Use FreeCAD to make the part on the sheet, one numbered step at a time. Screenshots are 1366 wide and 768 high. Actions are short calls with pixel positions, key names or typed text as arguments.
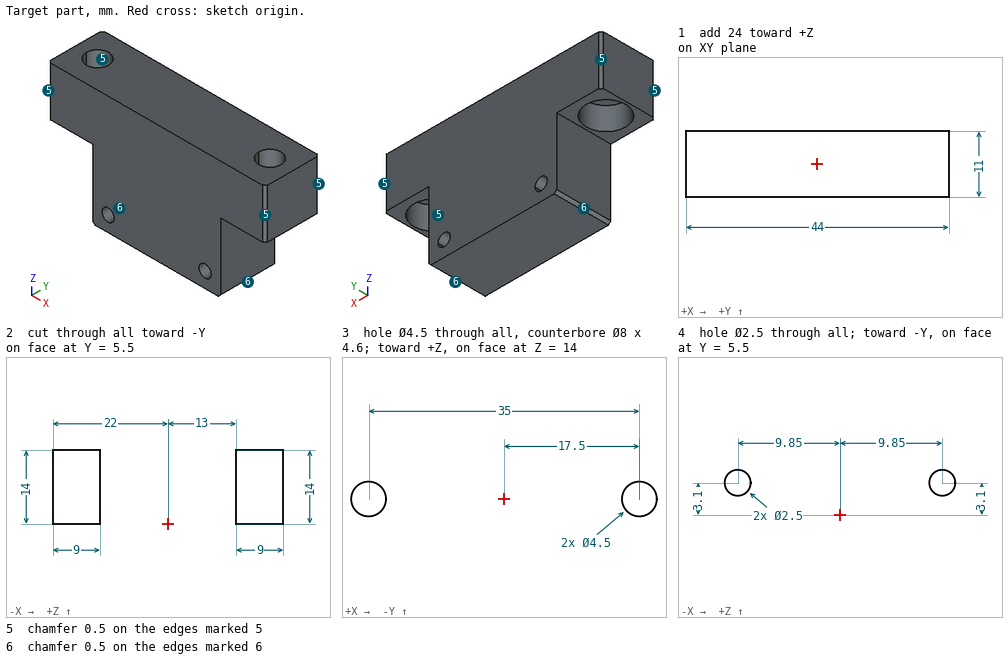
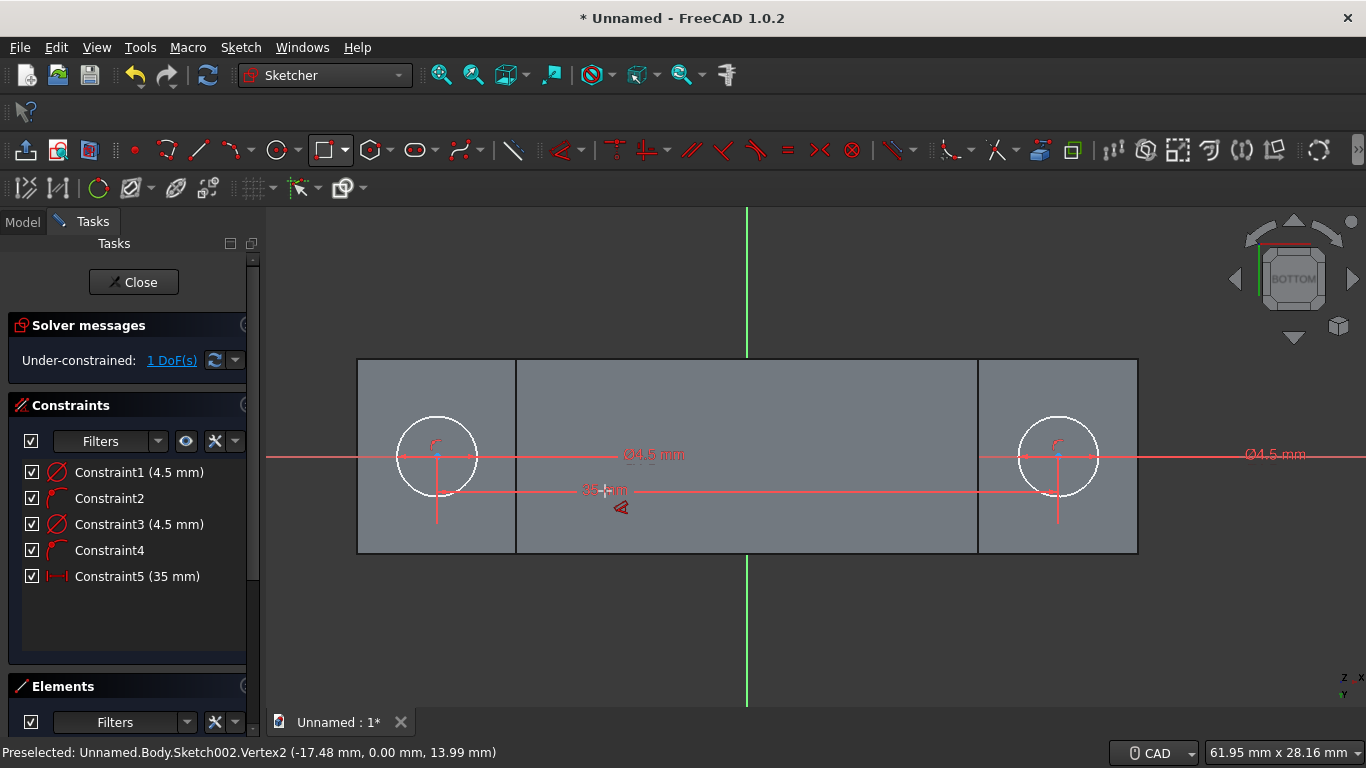
click(1058, 457)
click(903, 491)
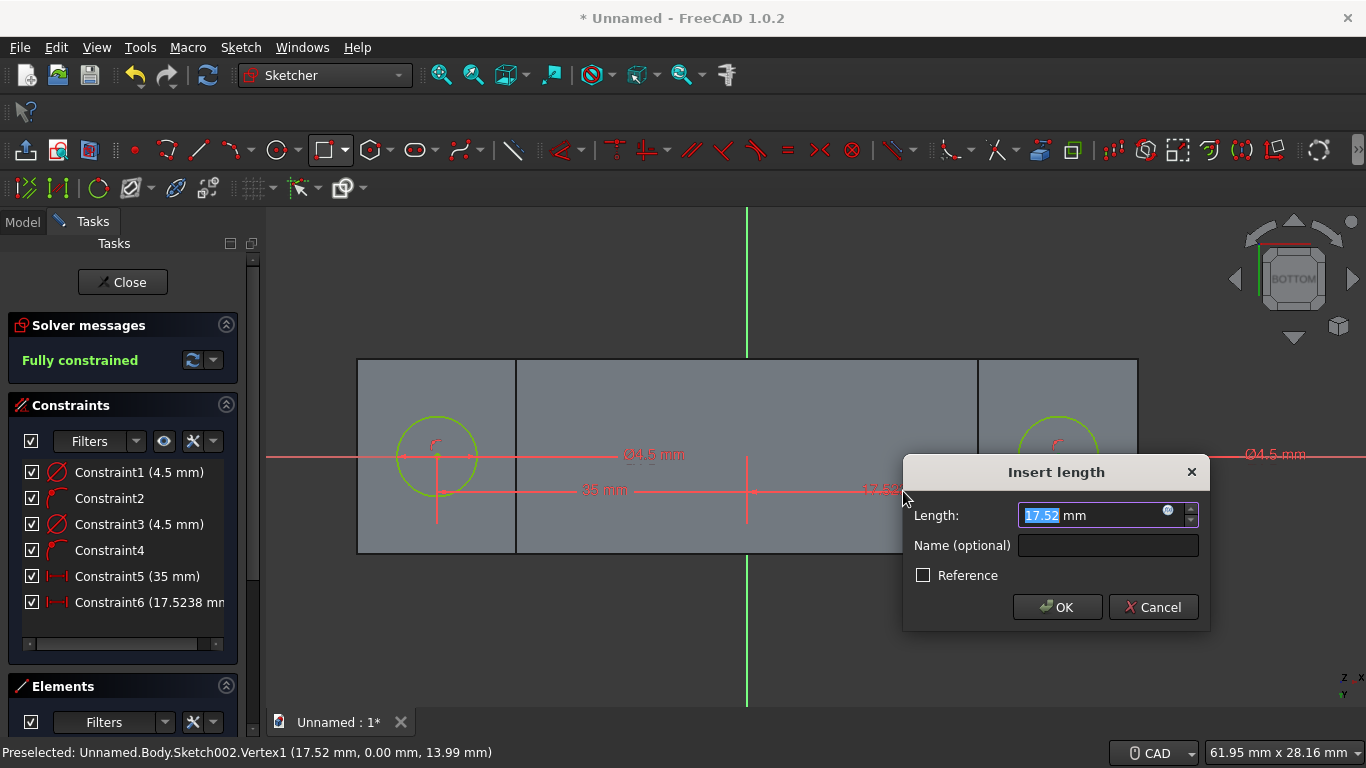
text(17.5)
key(Return)
key(Escape)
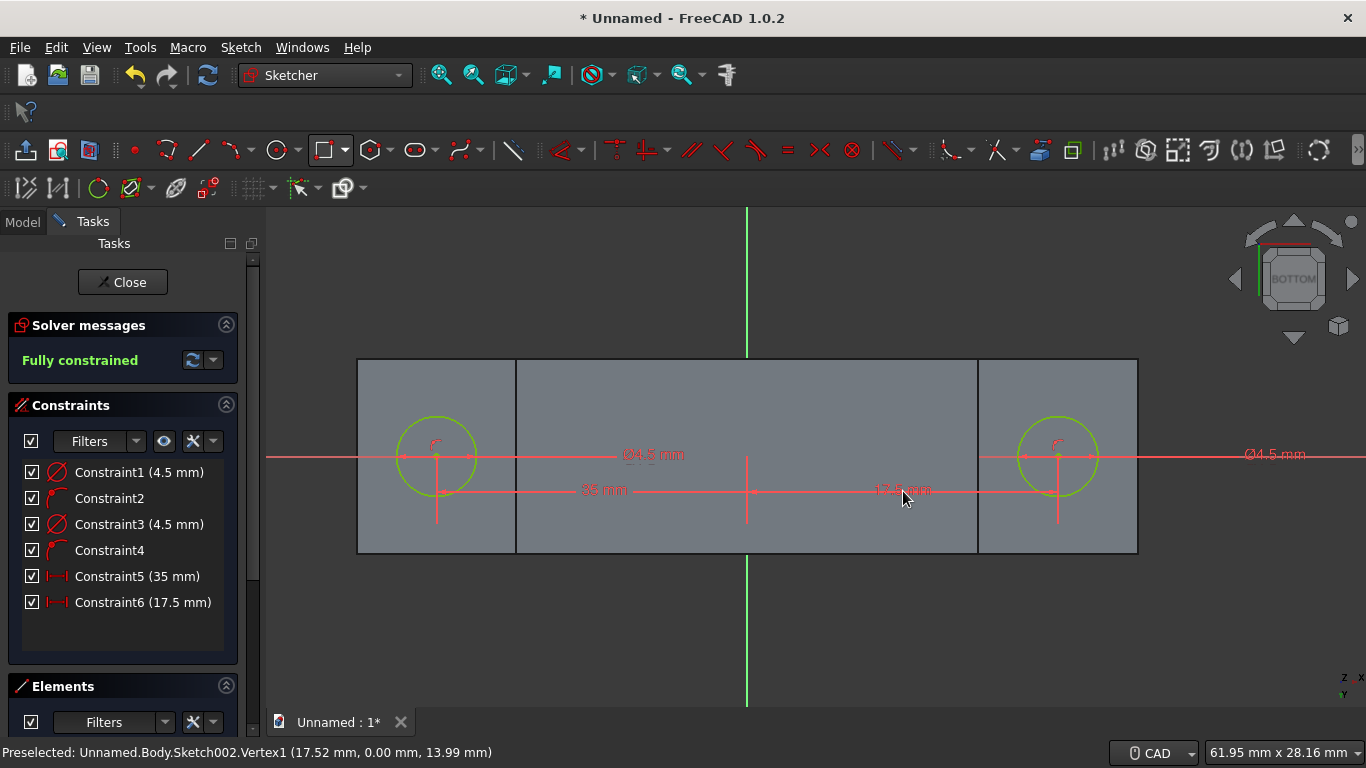
click(123, 282)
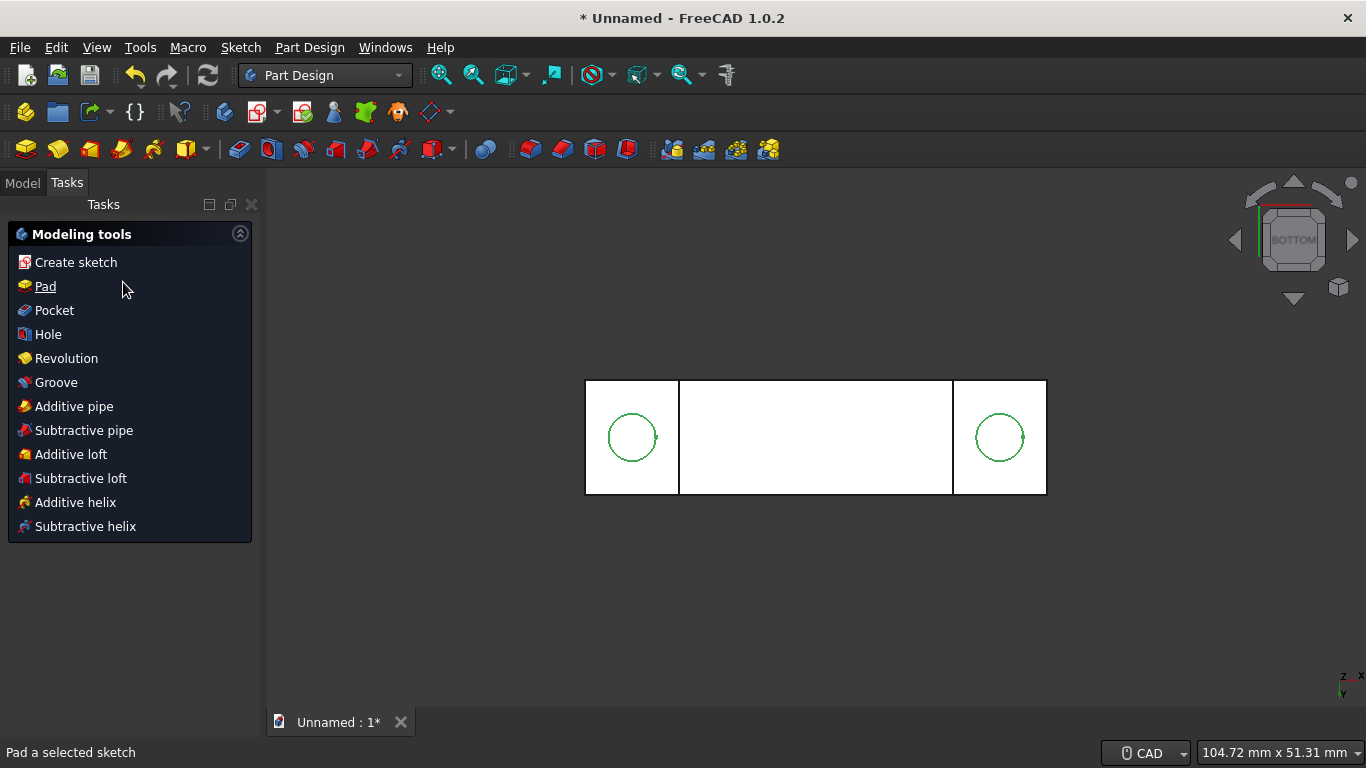
click(272, 150)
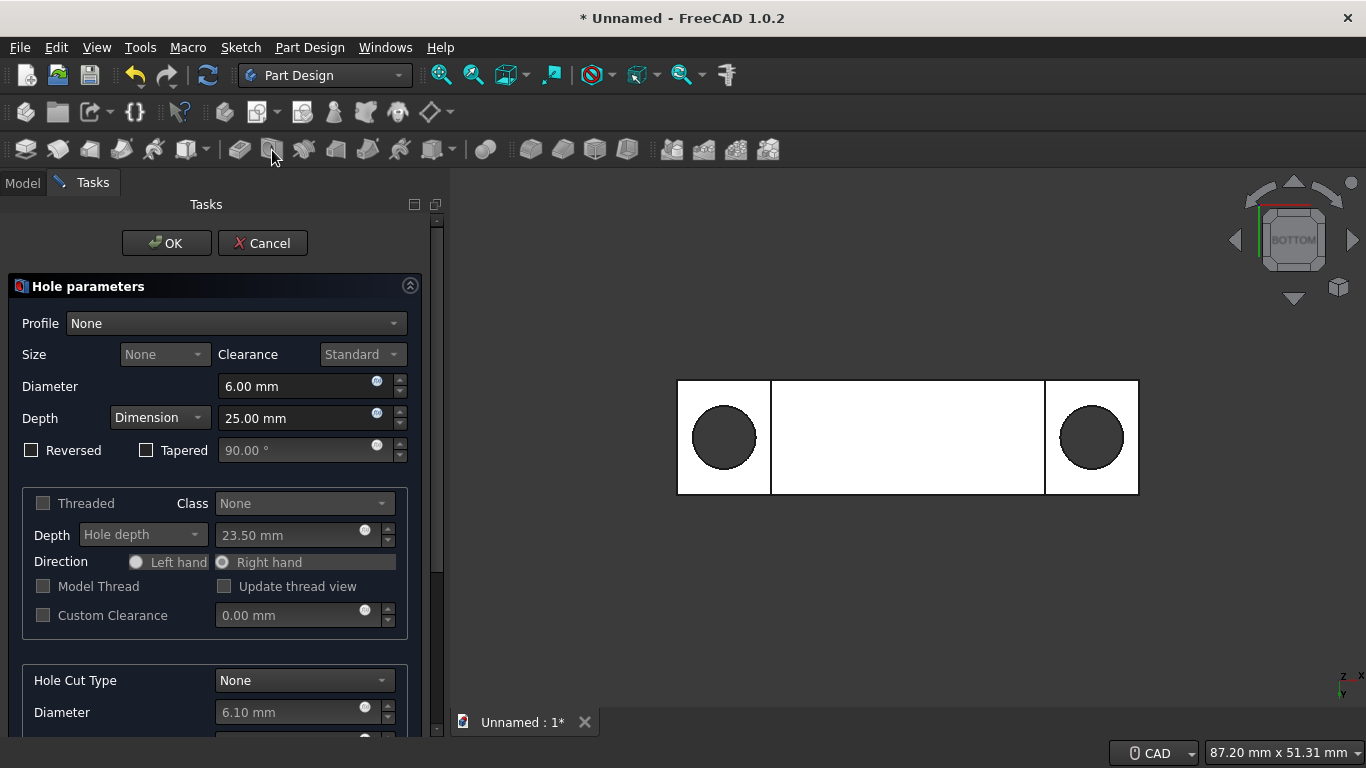
triple_click(305, 386)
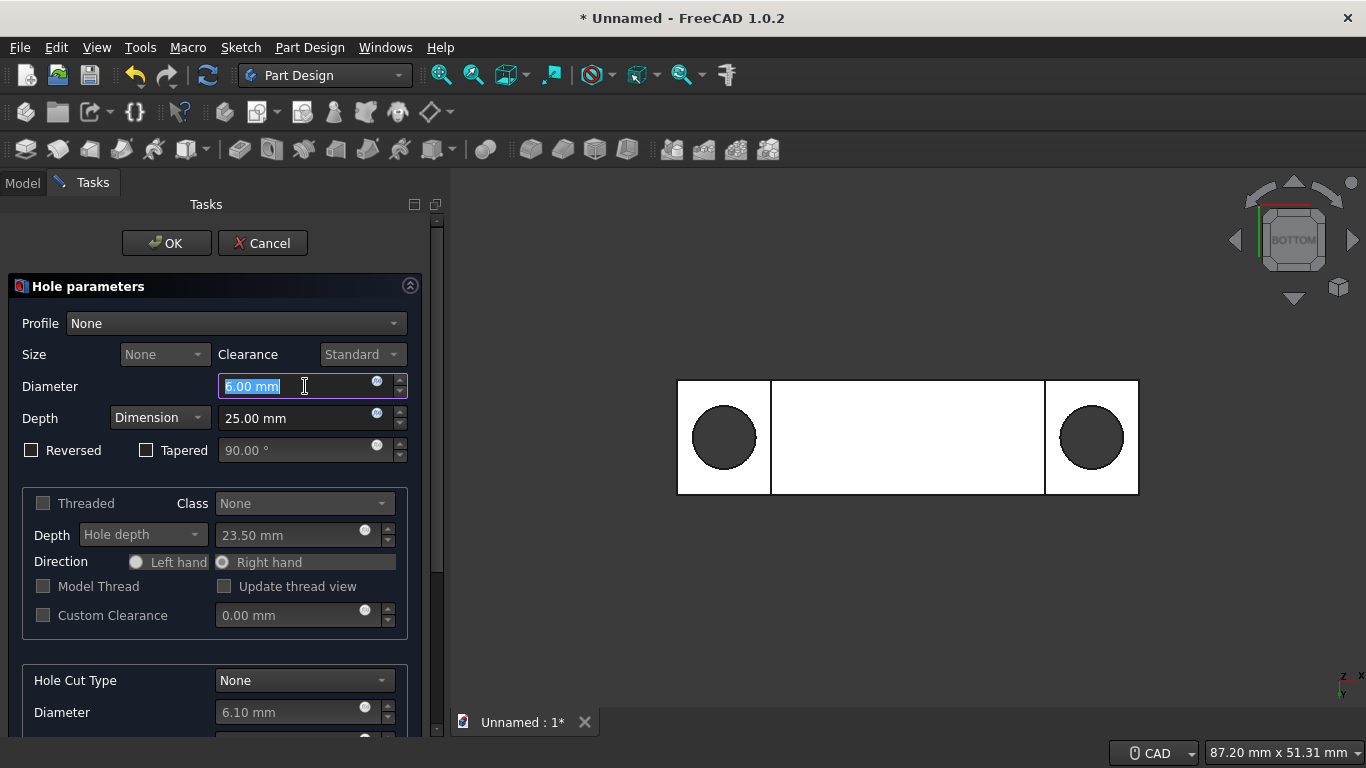
text(4.5)
key(Tab)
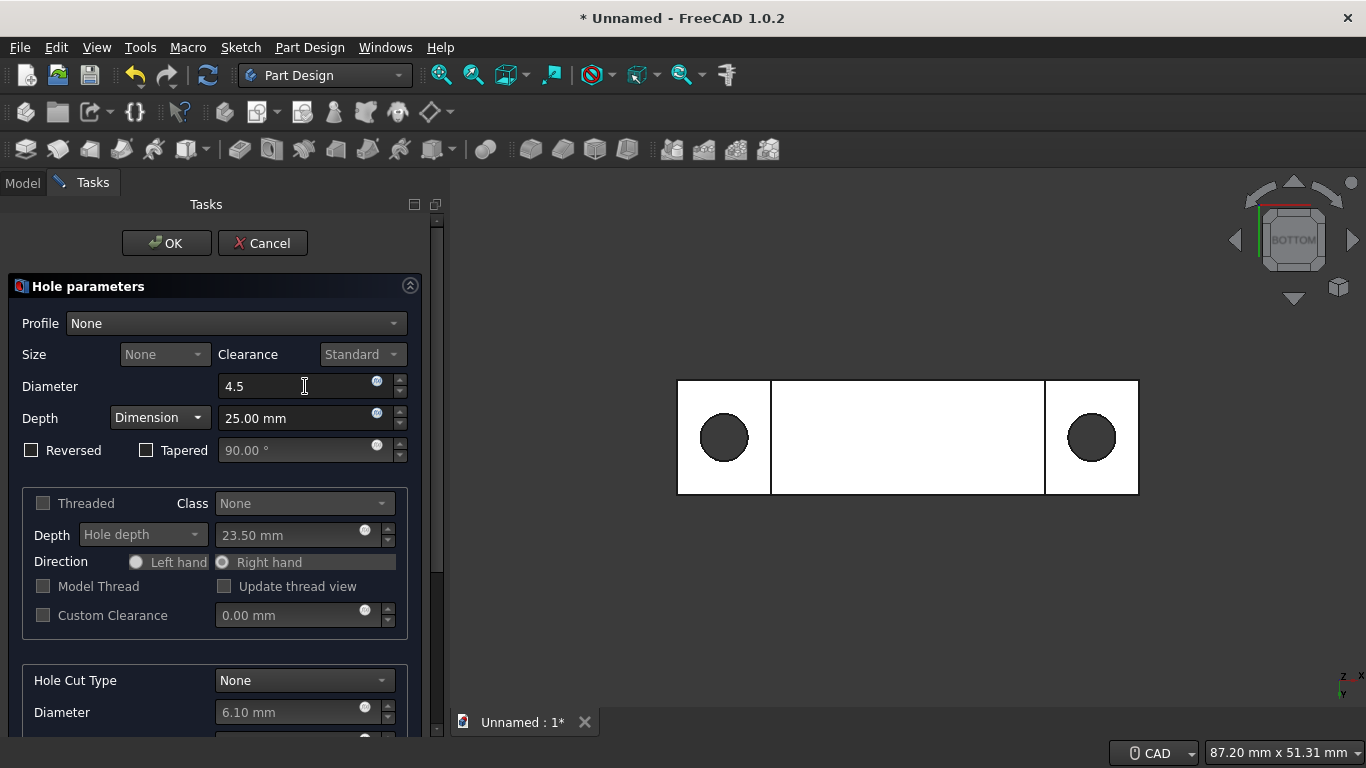
click(161, 418)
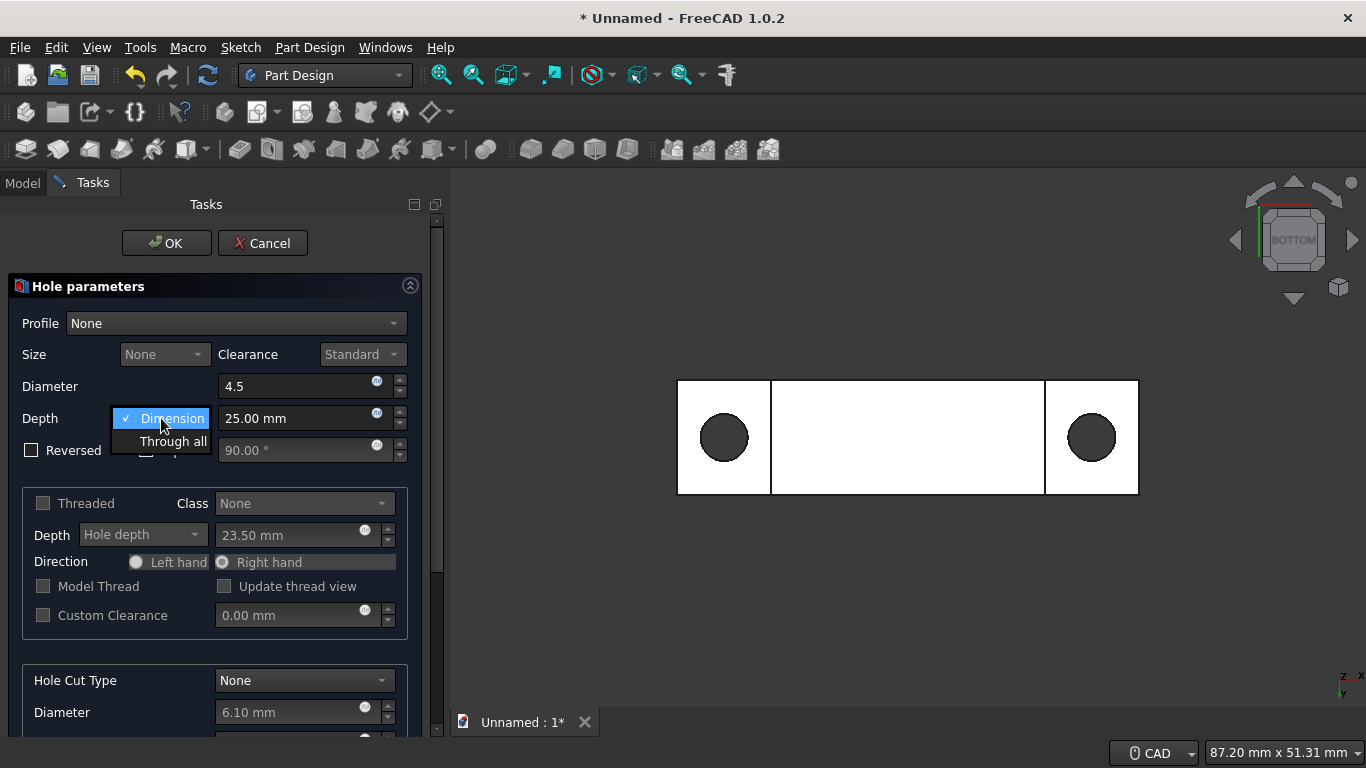
click(160, 442)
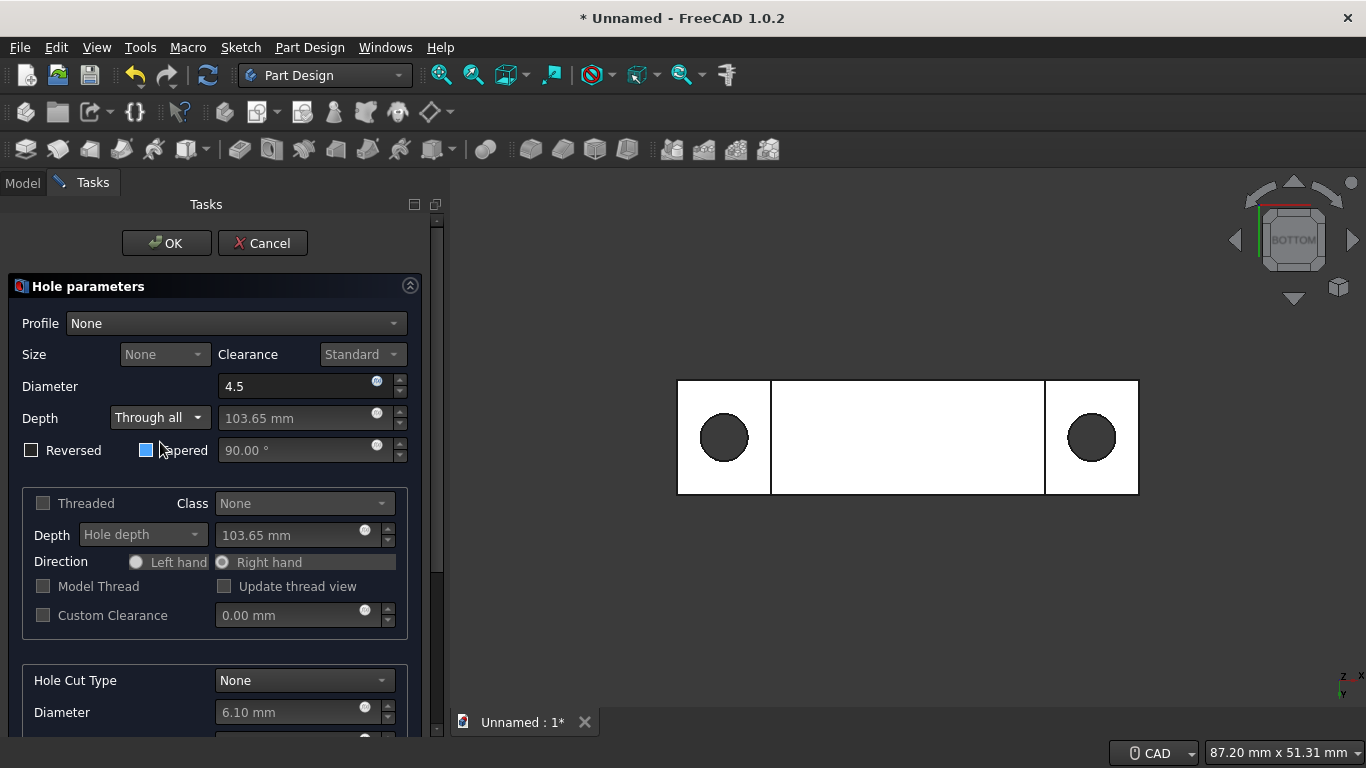
click(306, 680)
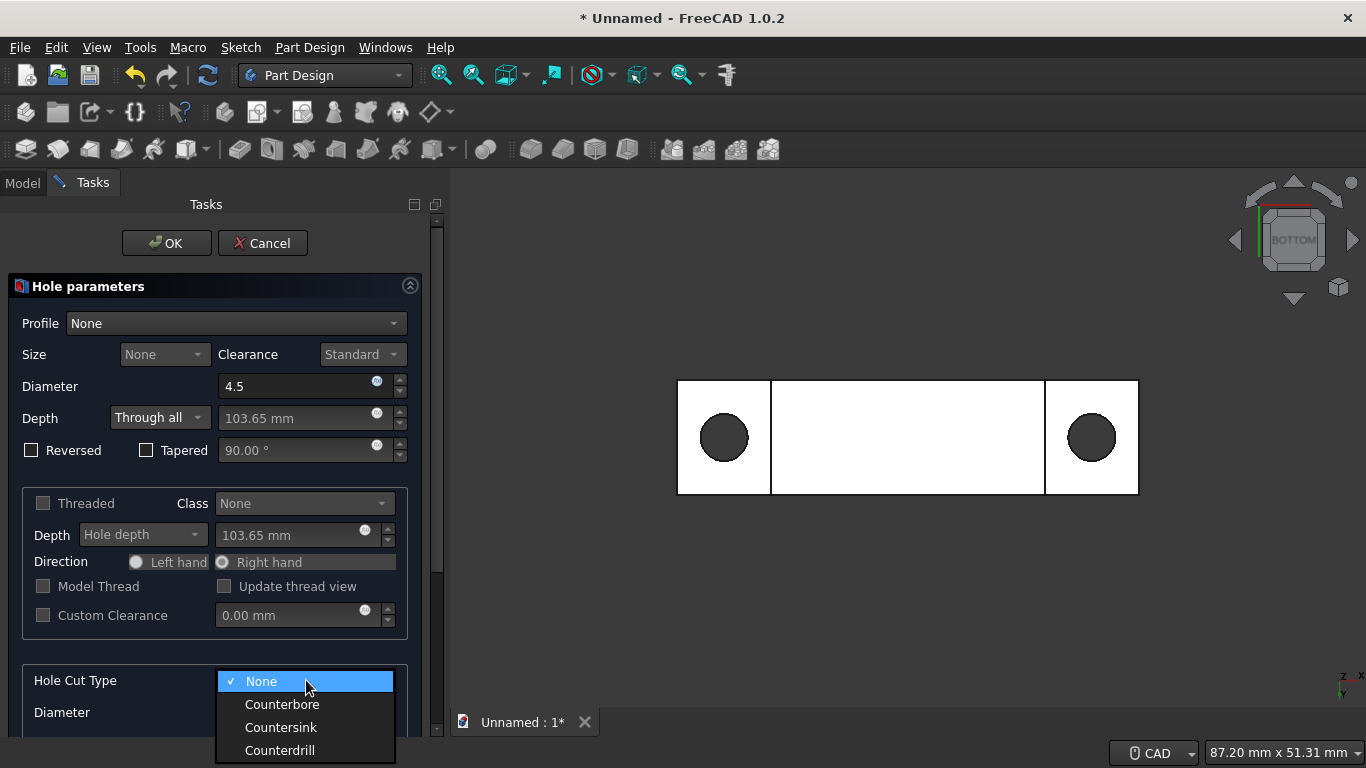
click(304, 704)